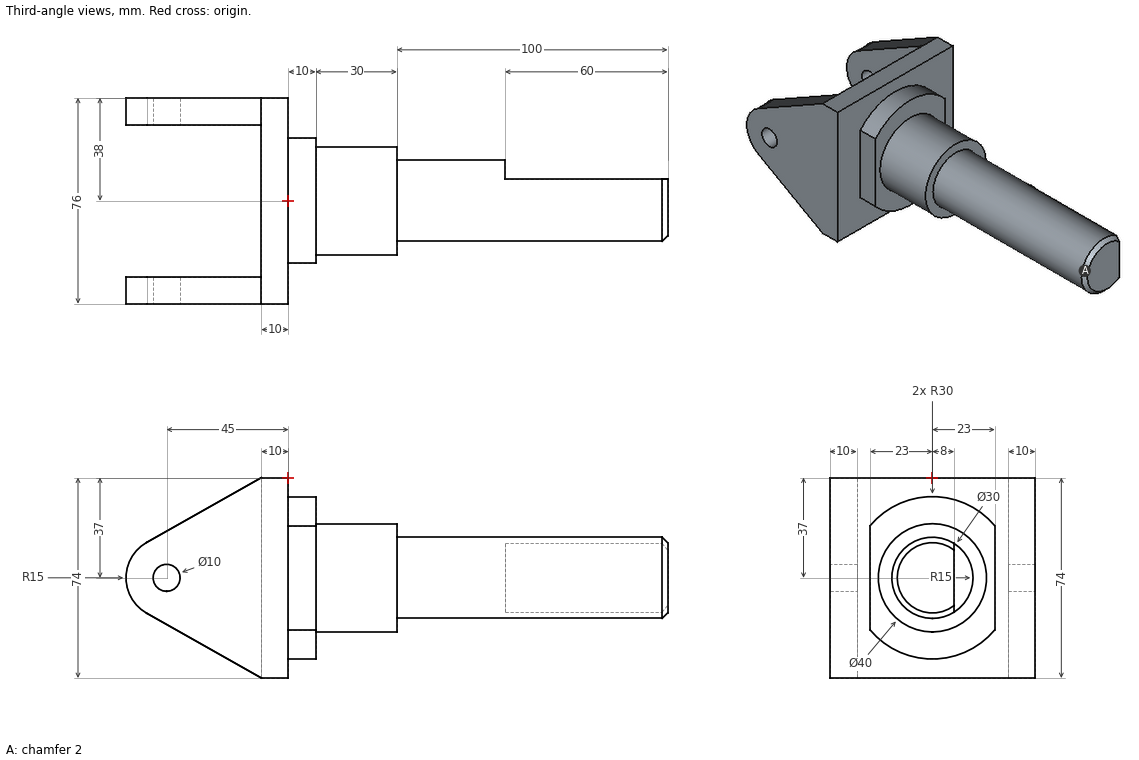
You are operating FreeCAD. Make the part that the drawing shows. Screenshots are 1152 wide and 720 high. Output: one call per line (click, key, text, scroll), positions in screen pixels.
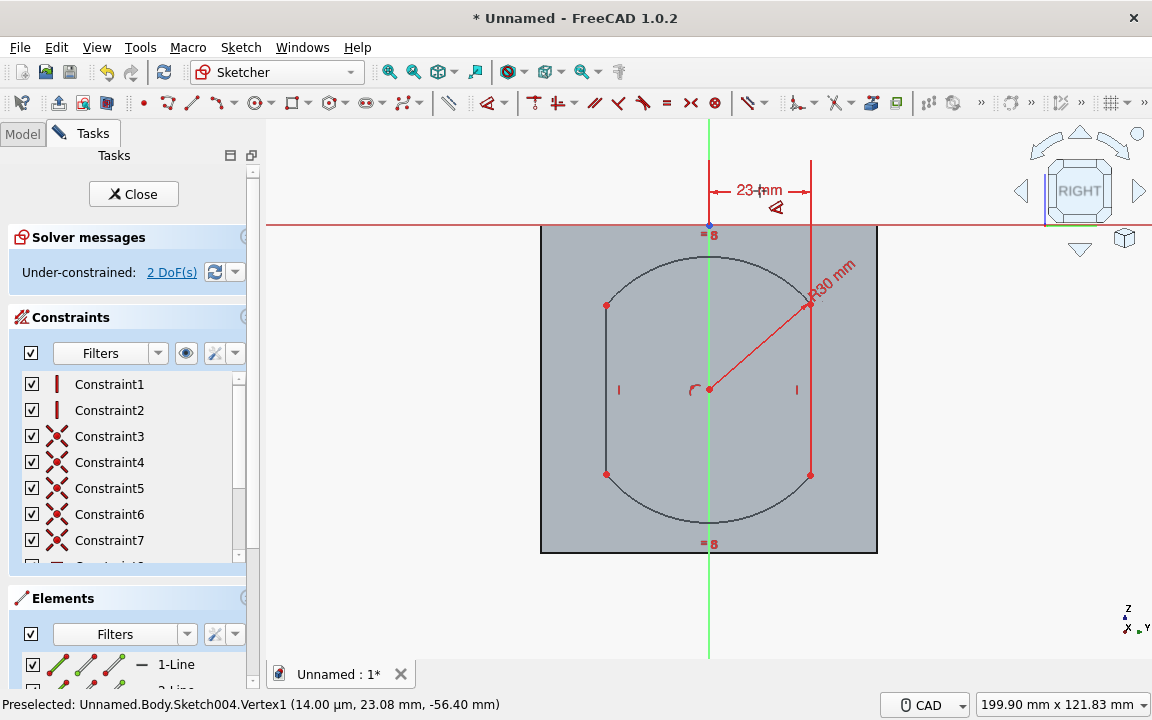
click(606, 305)
click(658, 191)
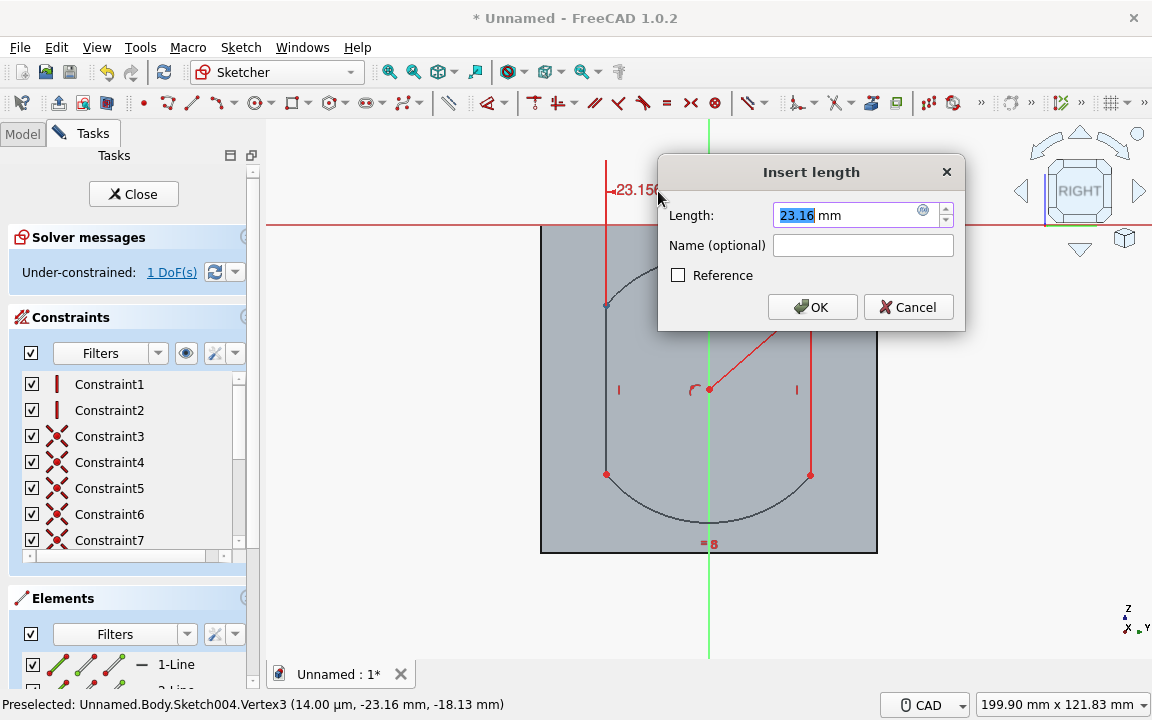
text(23)
key(Return)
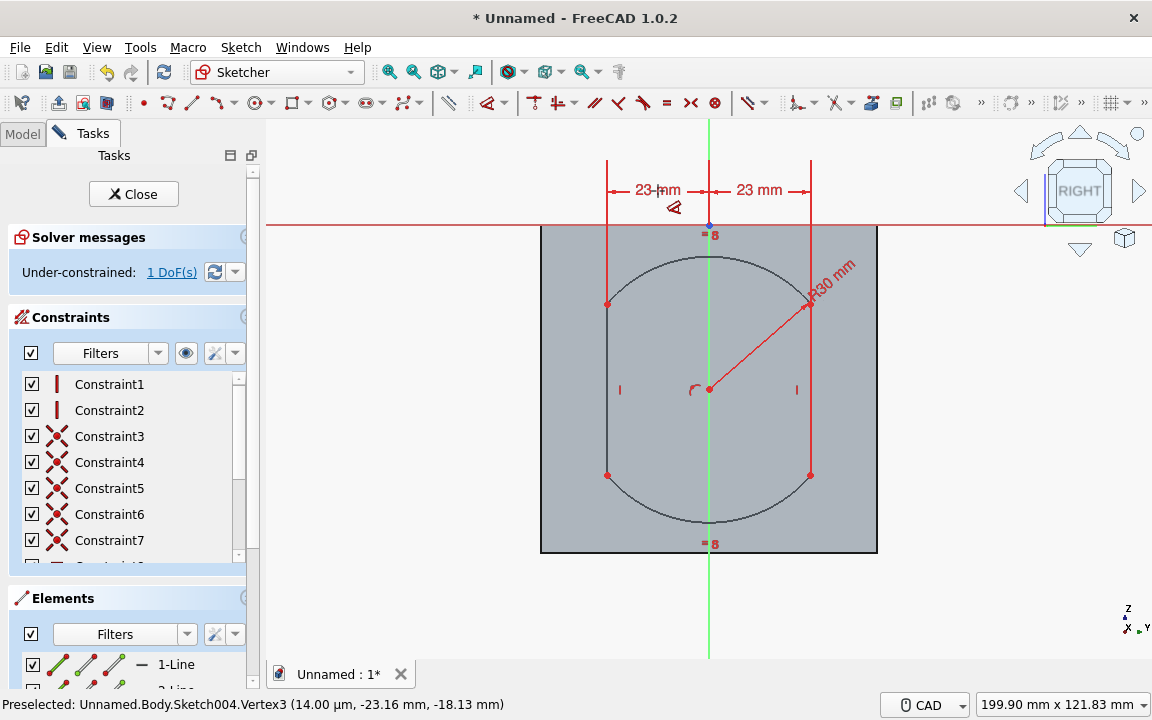
click(709, 390)
click(743, 307)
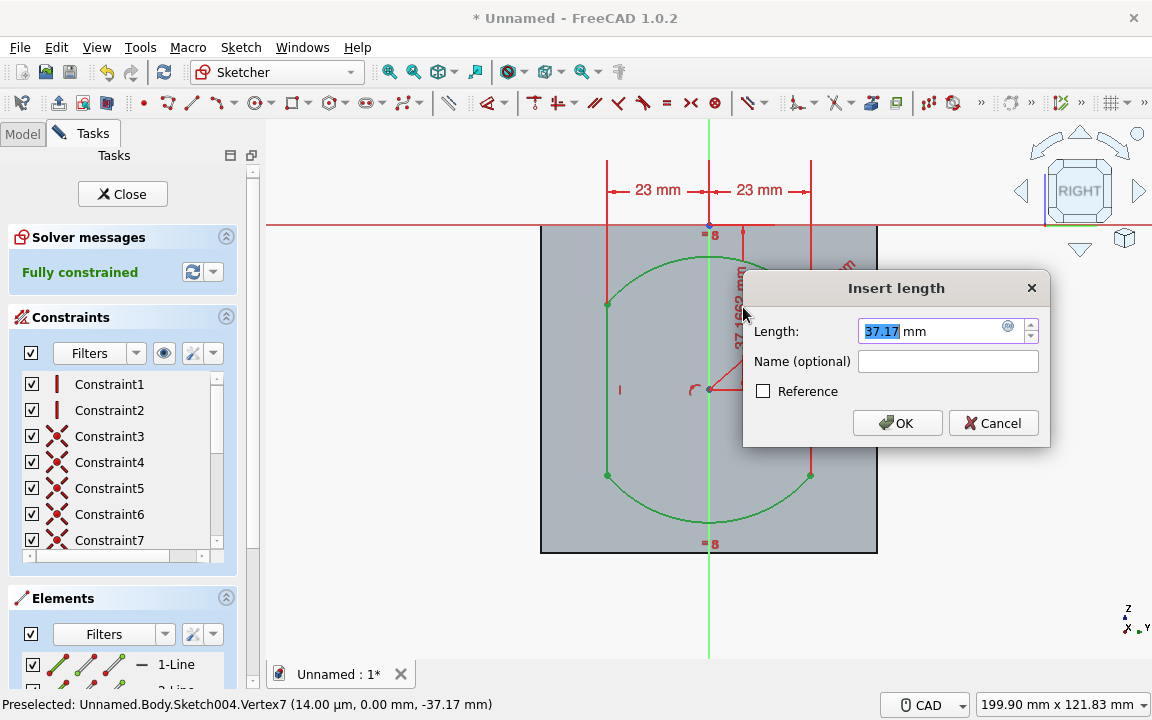
text(37)
key(Return)
key(Escape)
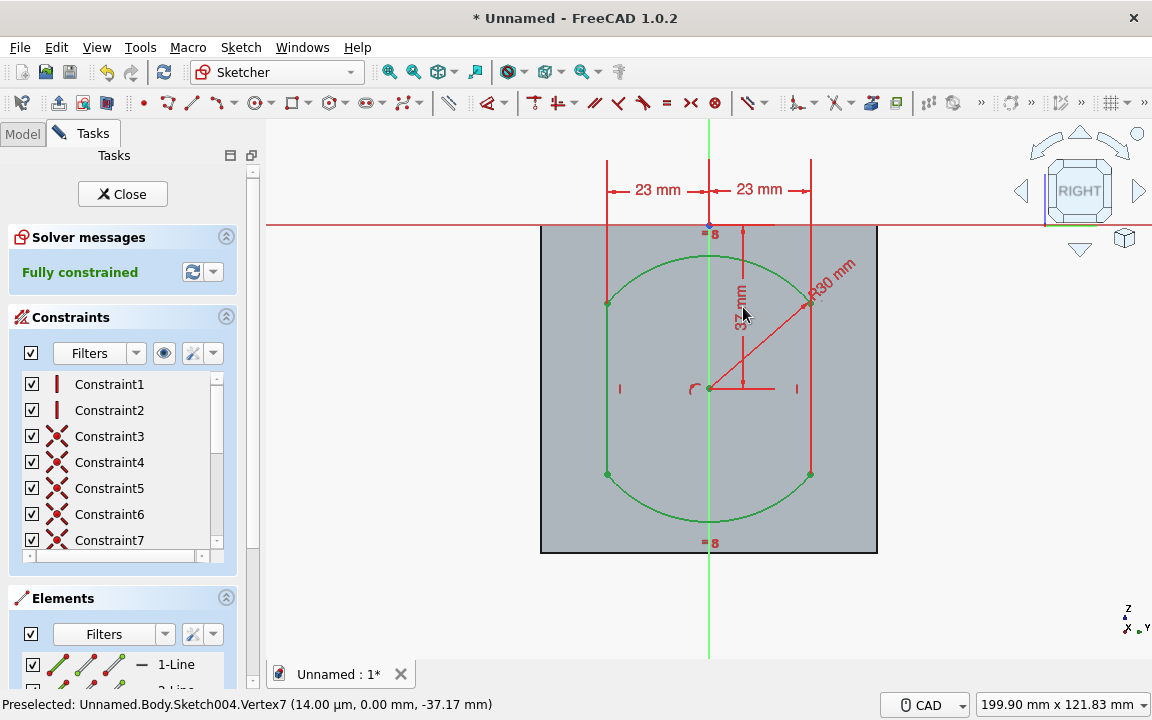
click(123, 194)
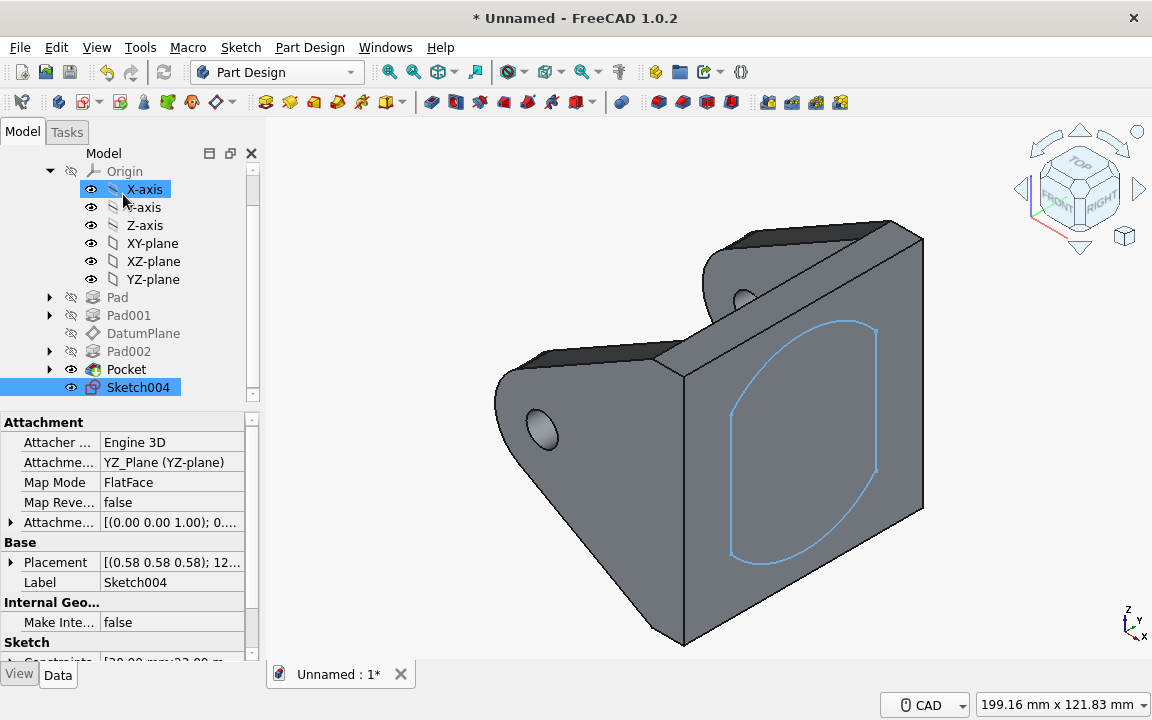
click(266, 102)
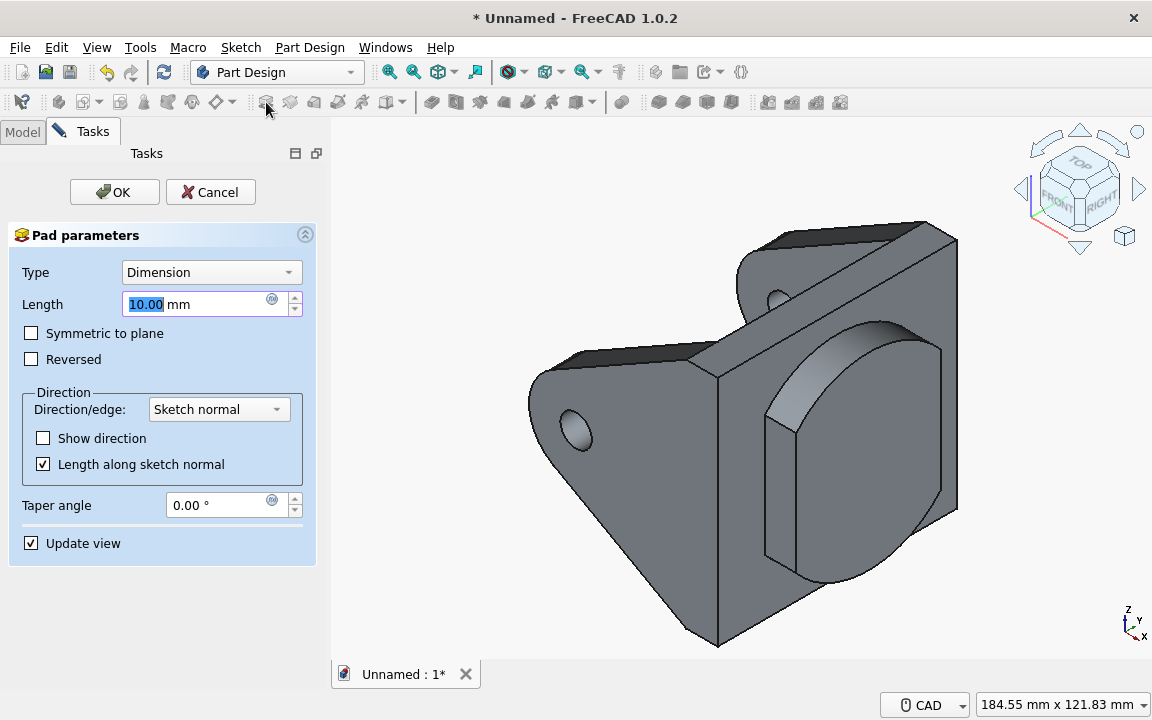
text(10)
key(Tab)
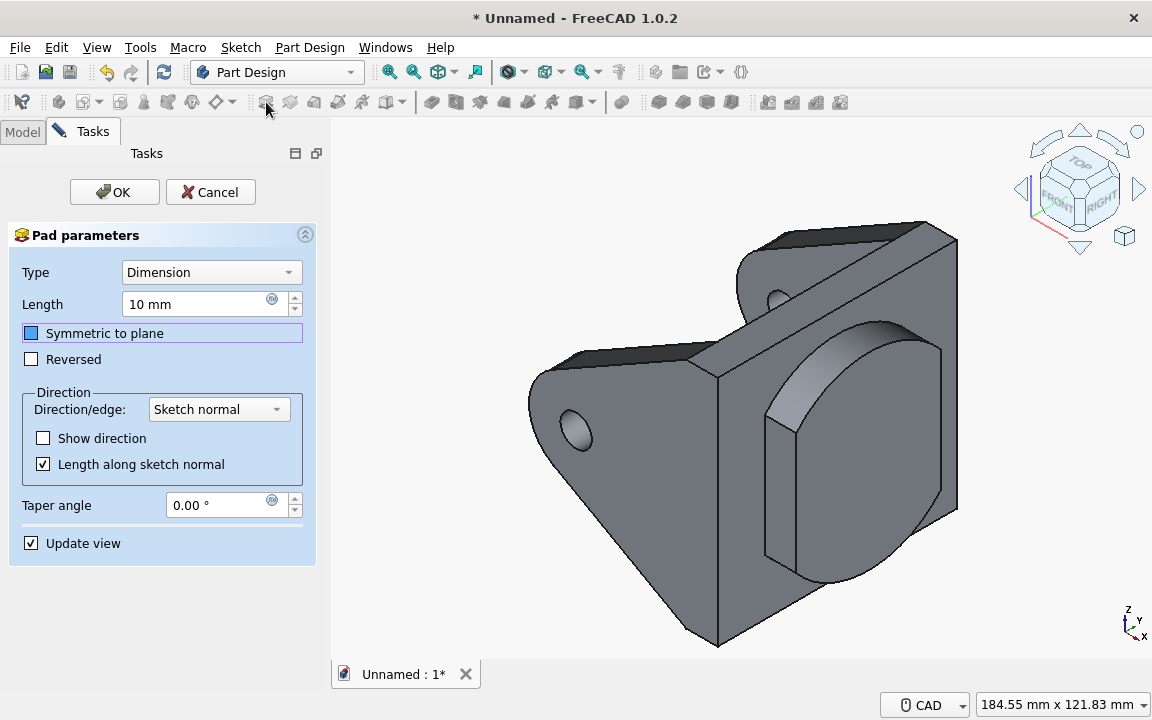
click(115, 192)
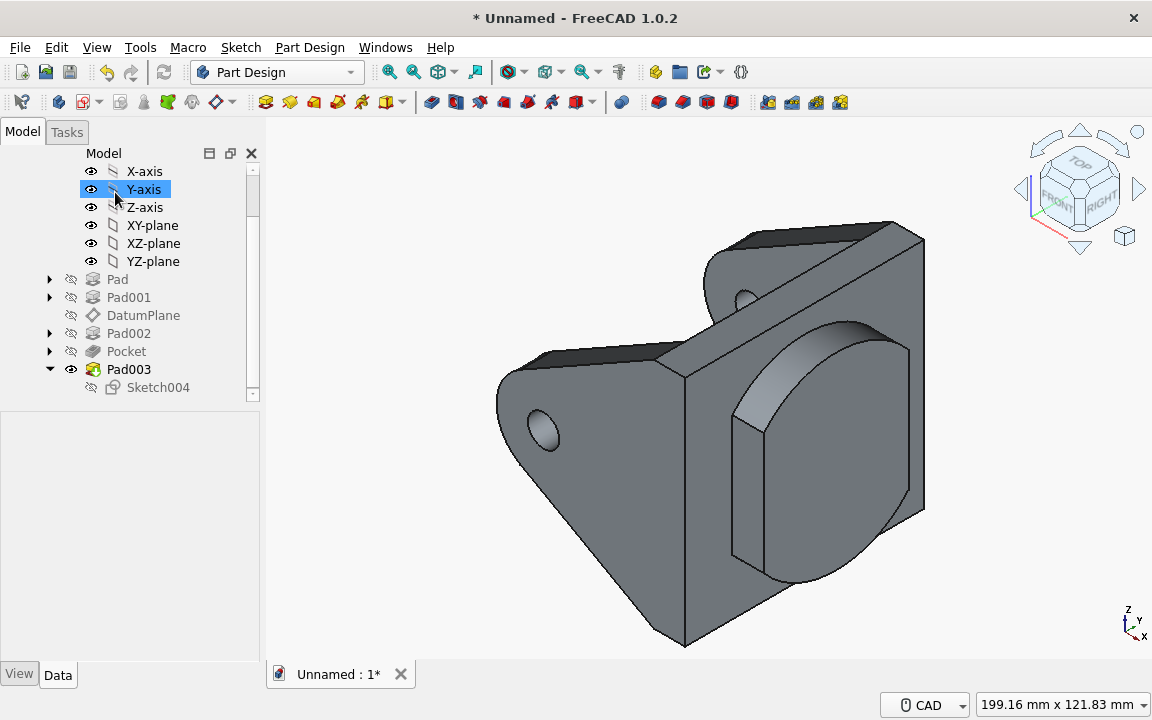
click(390, 72)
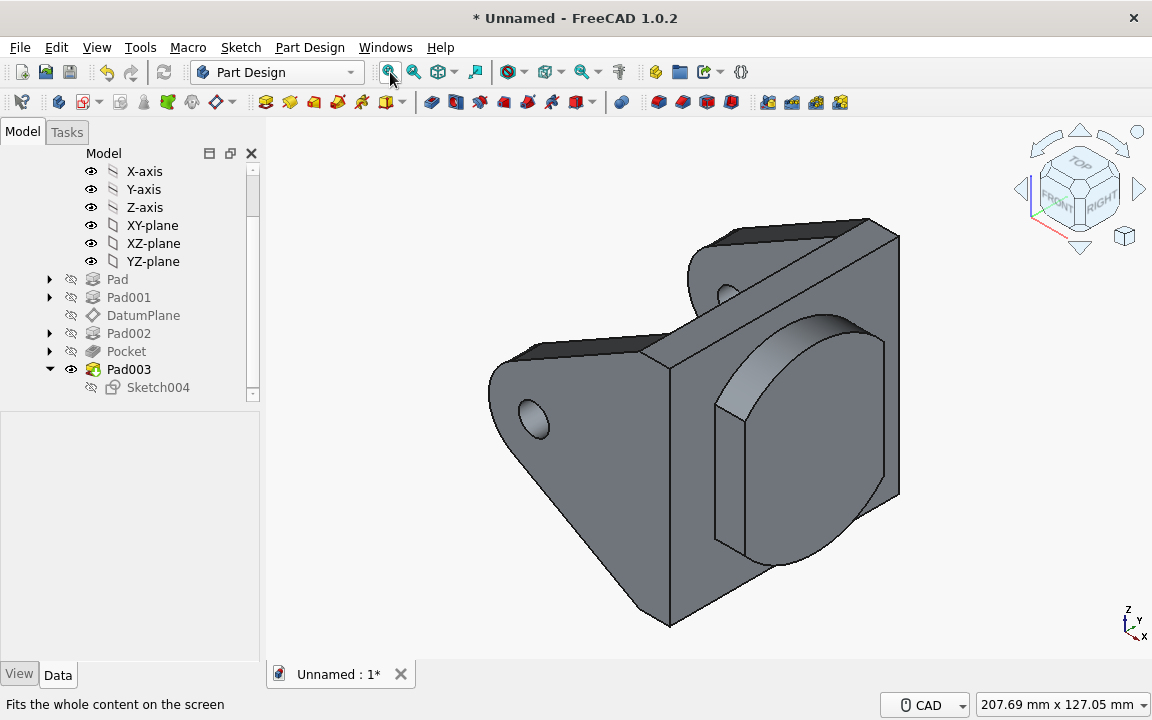
click(814, 448)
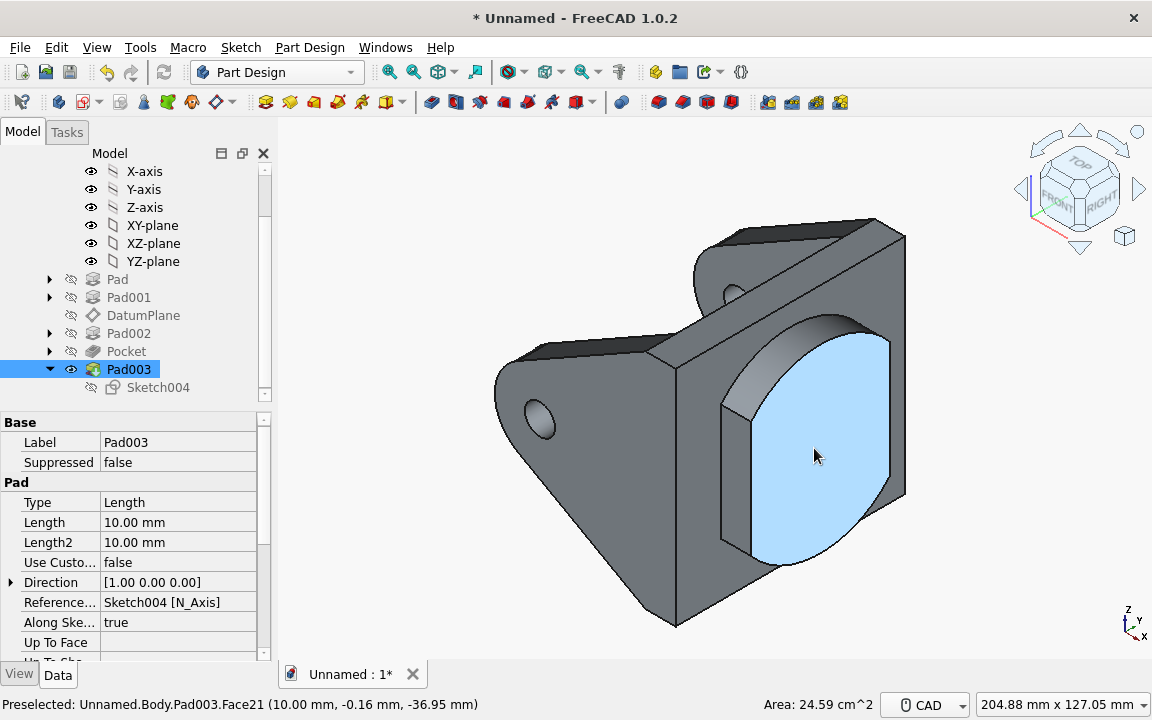
click(84, 102)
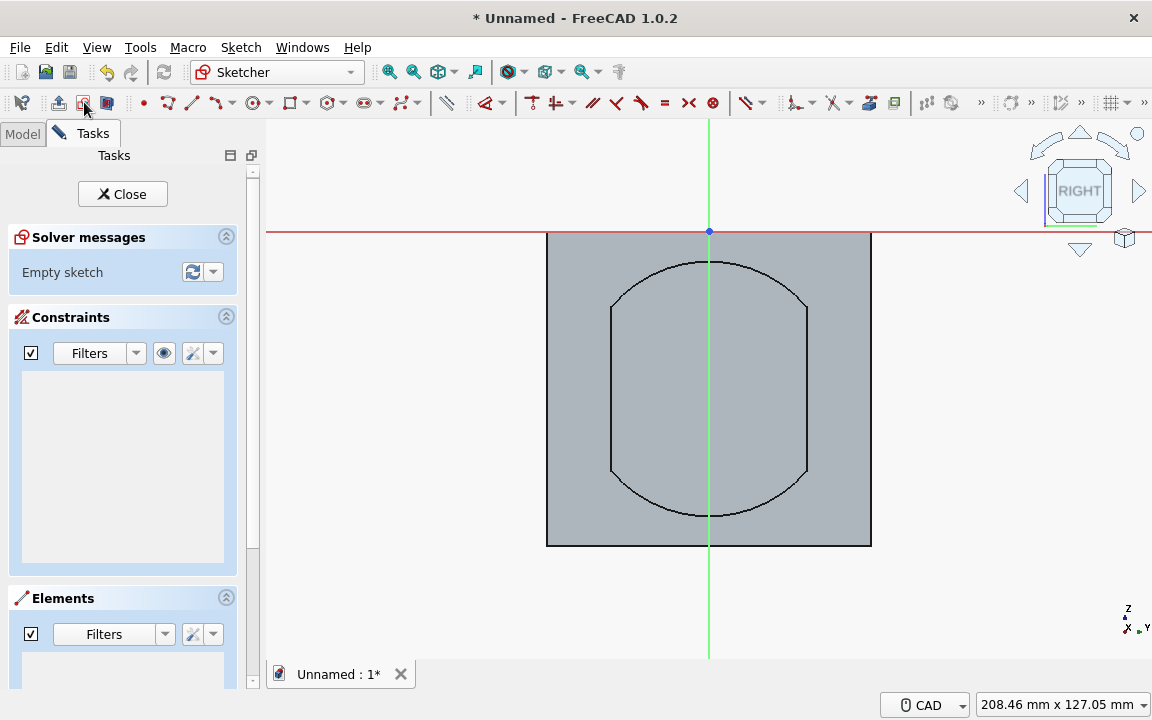
scroll(848, 279, up, 2)